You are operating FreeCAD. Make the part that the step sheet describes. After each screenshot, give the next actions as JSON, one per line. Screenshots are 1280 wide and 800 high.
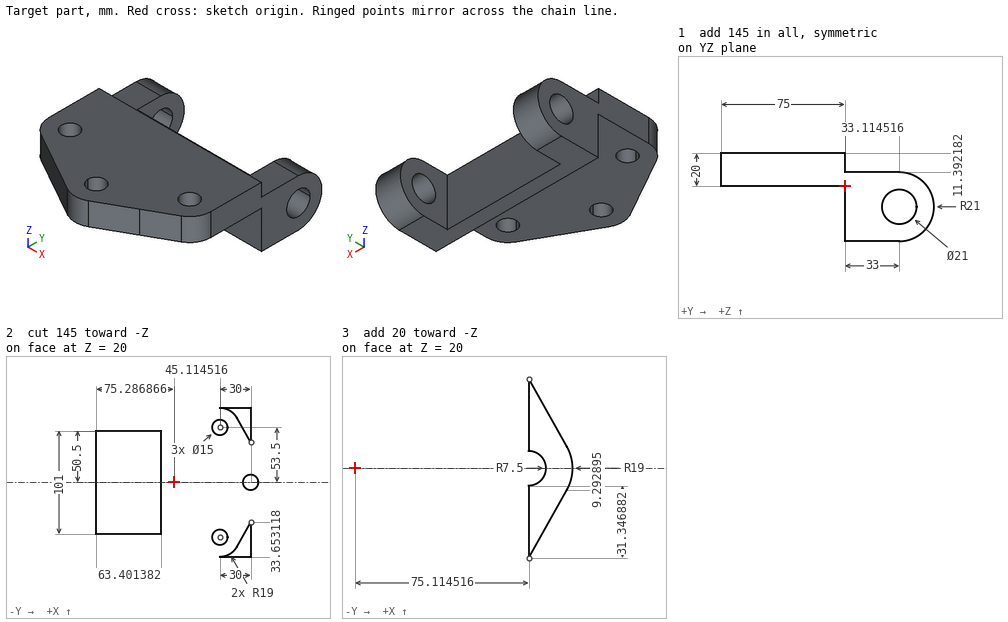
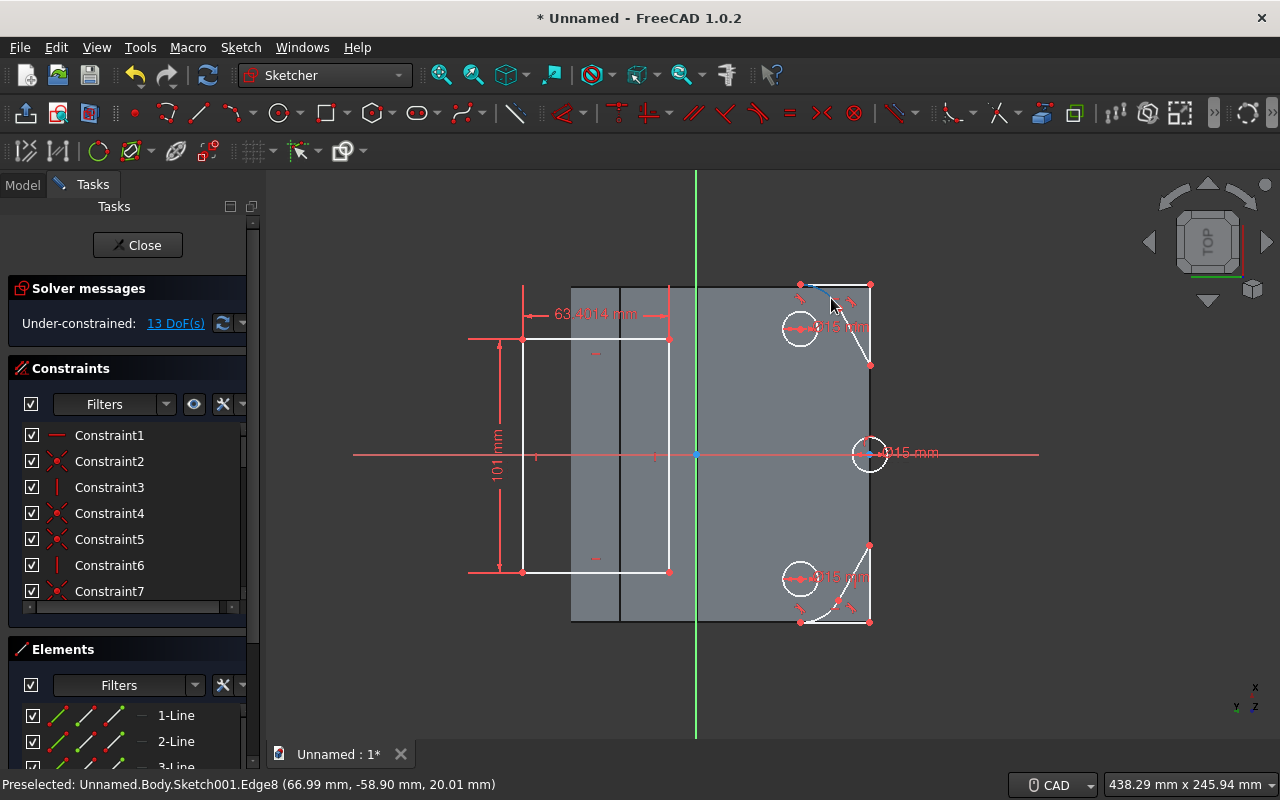
{"action": "scroll", "coordinate": [830, 611], "scroll_direction": "up", "scroll_amount": 4}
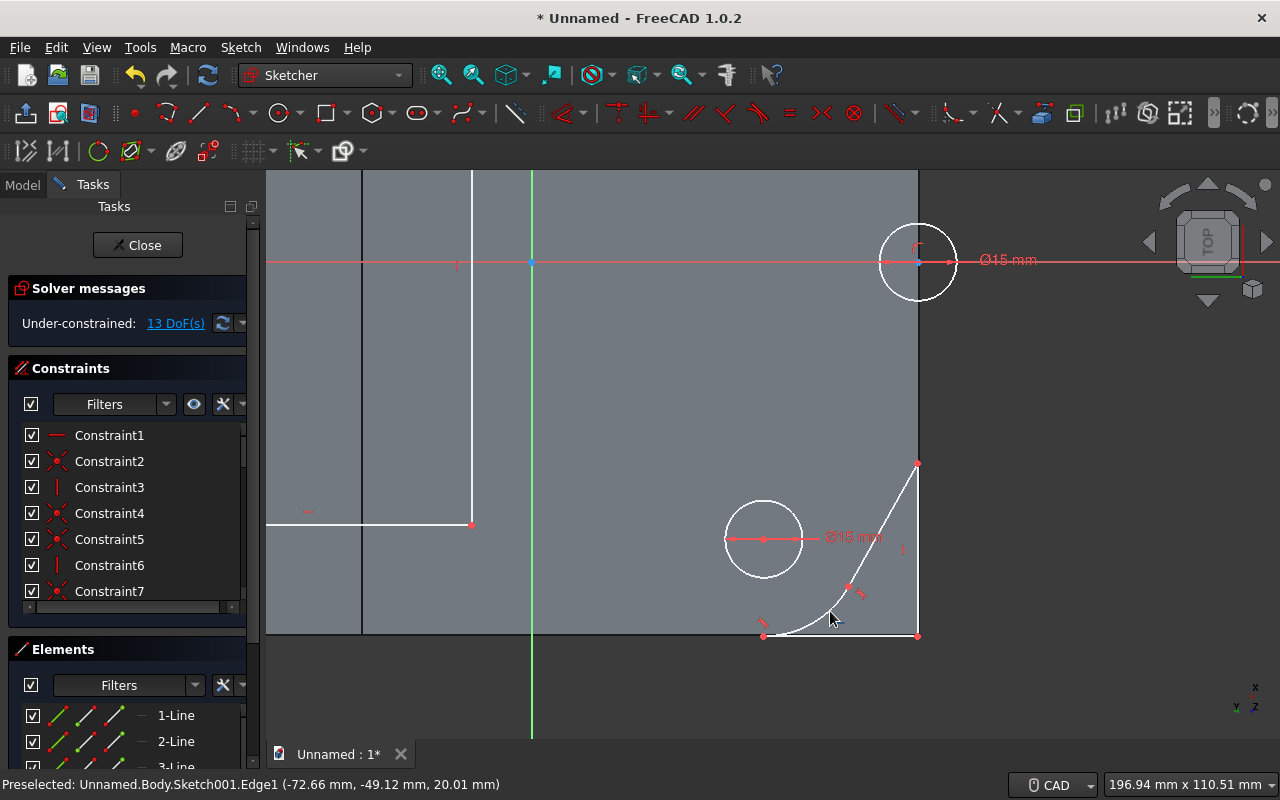
{"action": "left_click", "coordinate": [830, 611]}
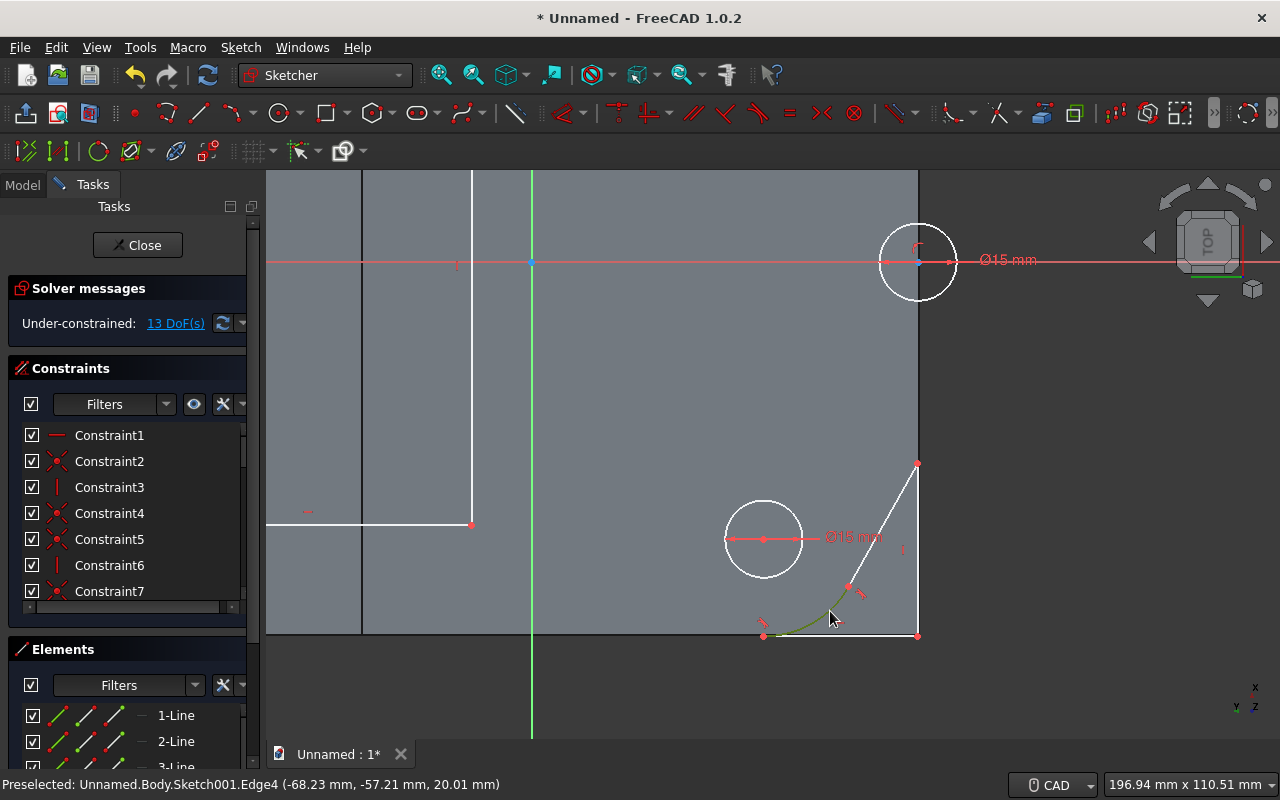
{"action": "scroll", "coordinate": [830, 611], "scroll_direction": "down", "scroll_amount": 4}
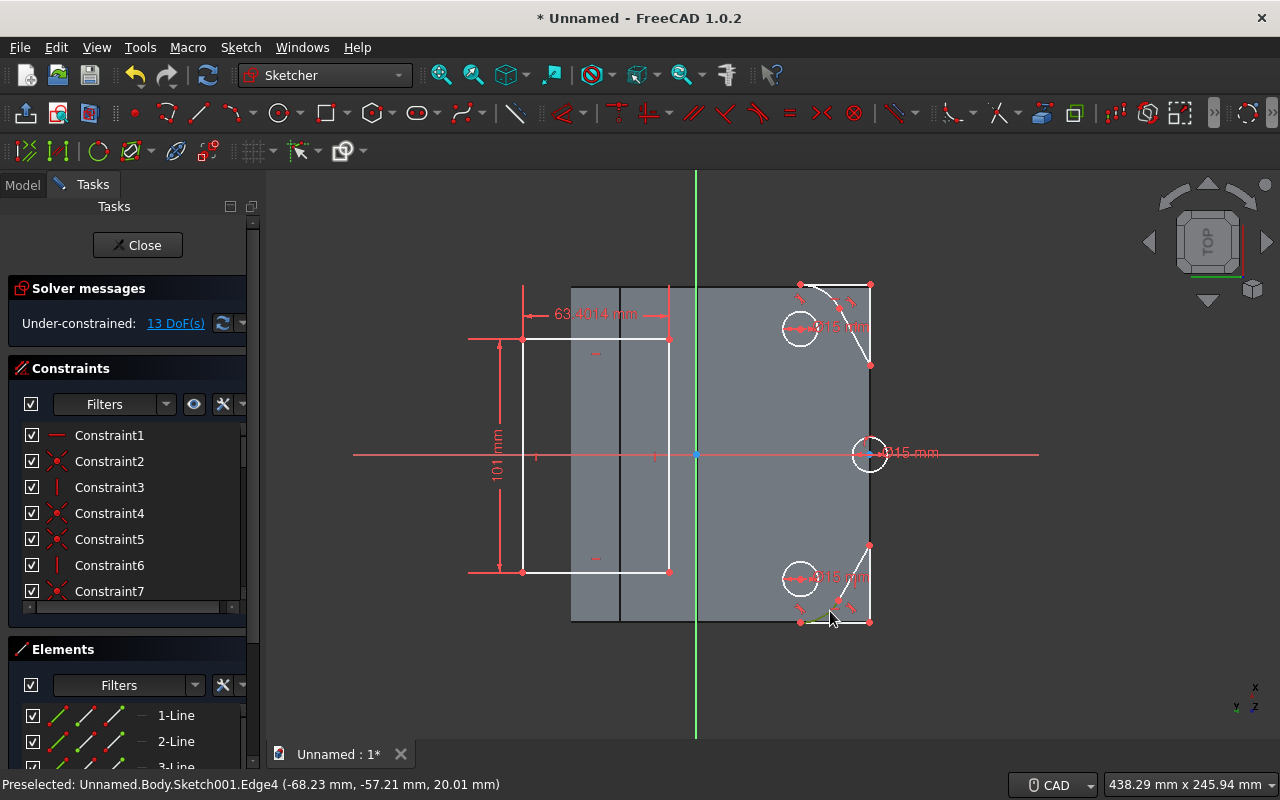
{"action": "left_click", "coordinate": [823, 291]}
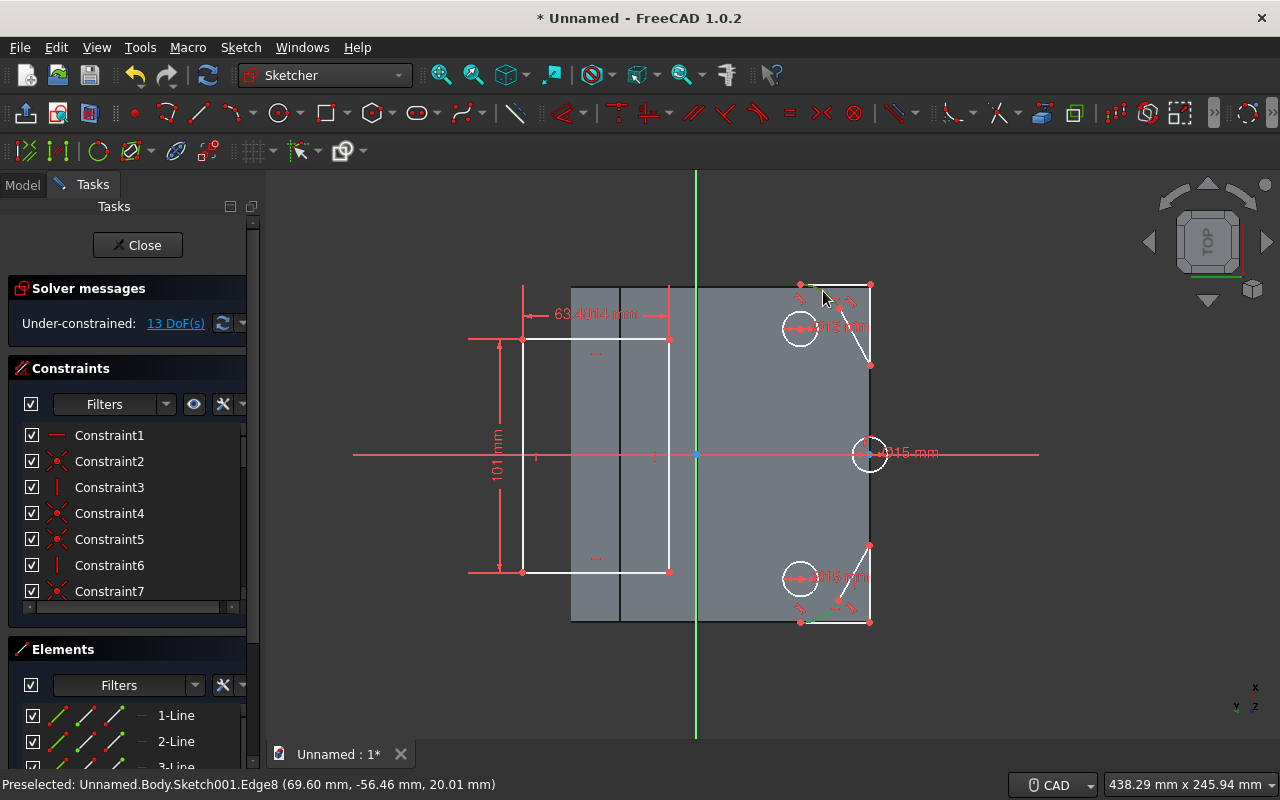
{"action": "left_click", "coordinate": [790, 114]}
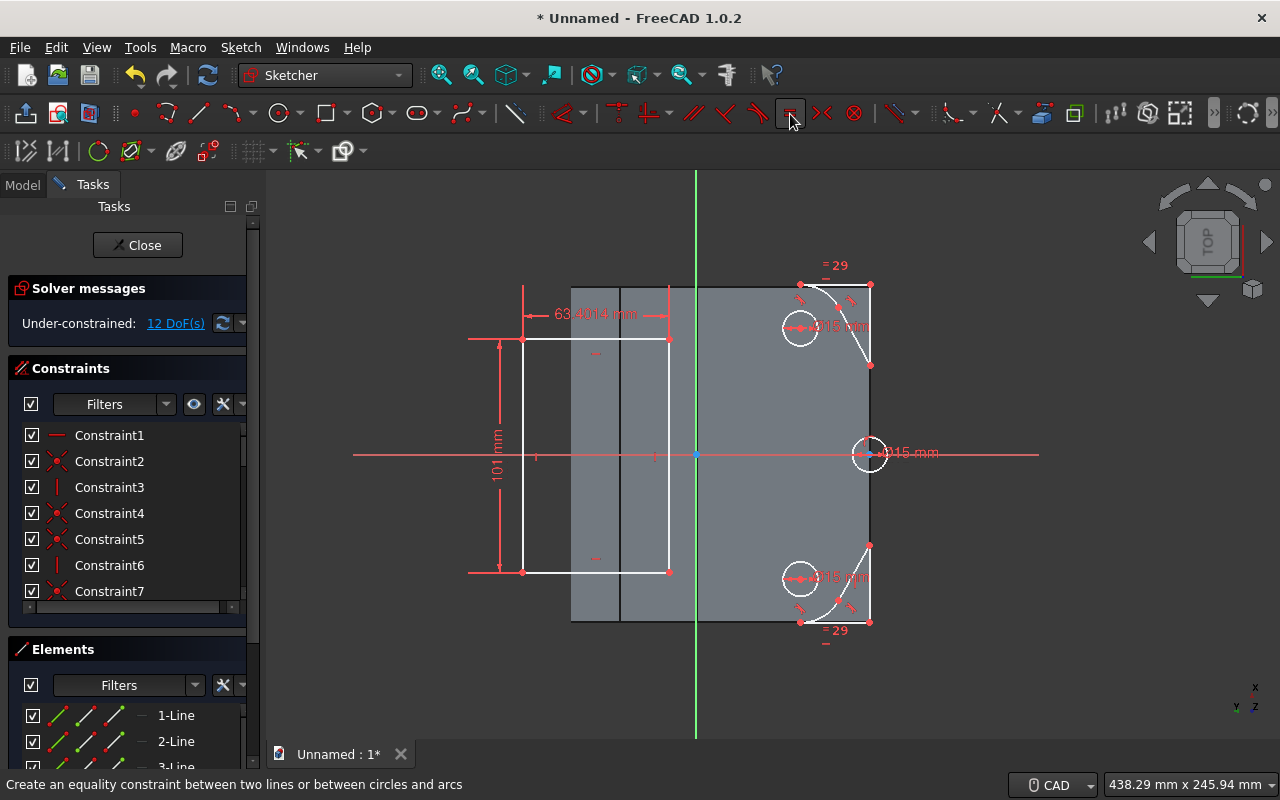
{"action": "left_click", "coordinate": [801, 579]}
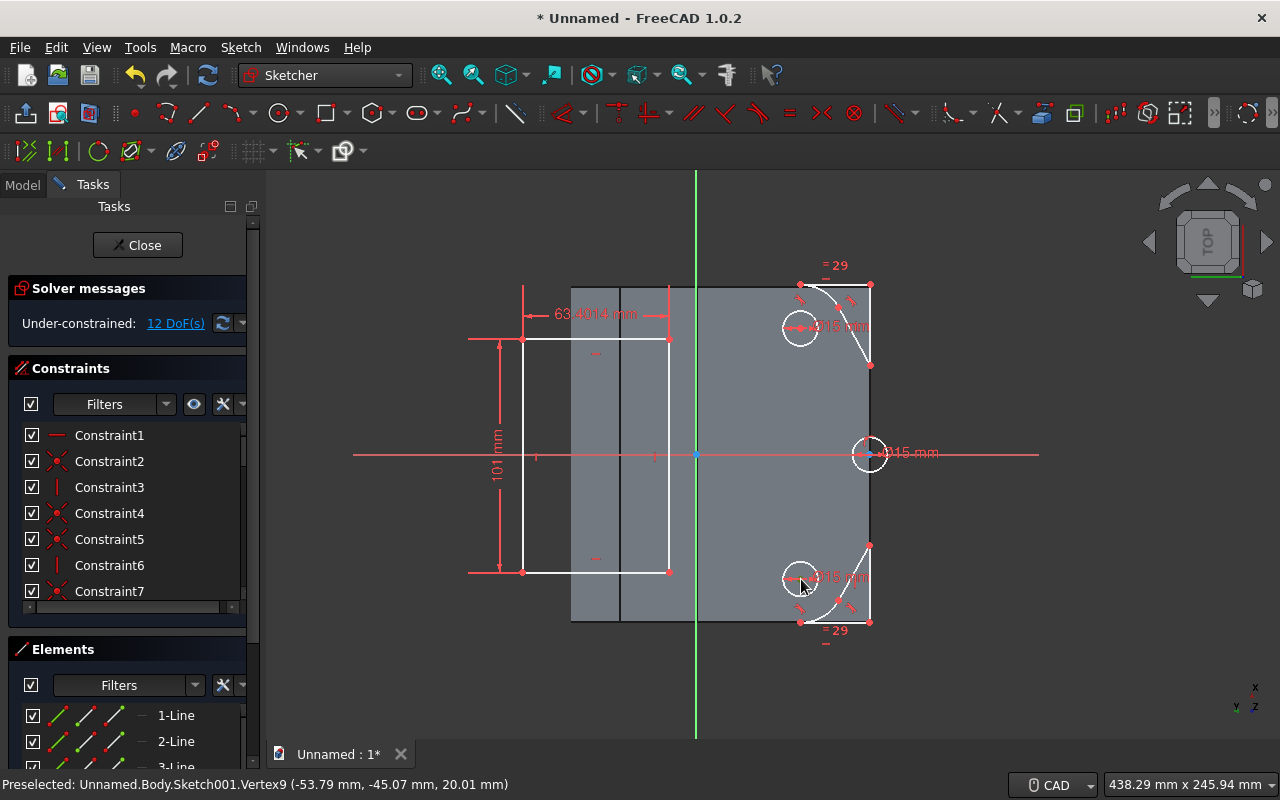
{"action": "left_click", "coordinate": [800, 328]}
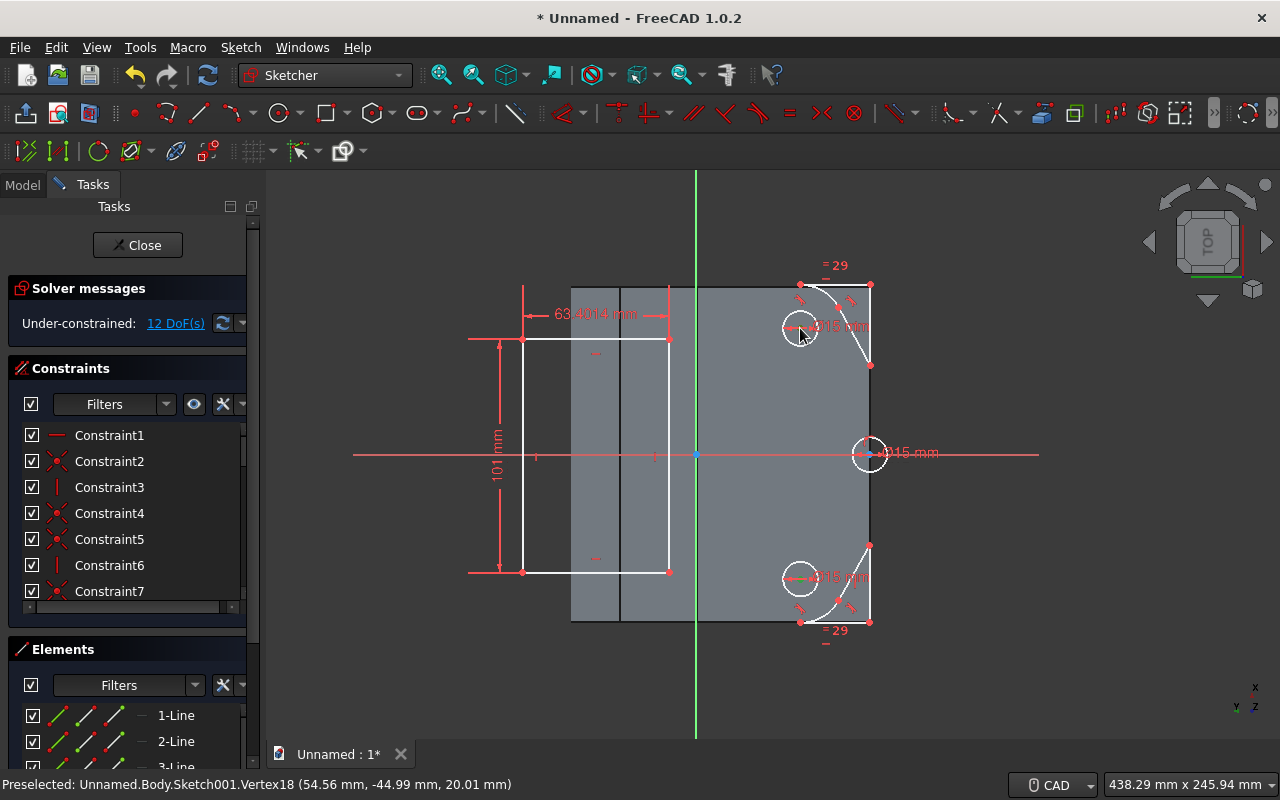
{"action": "left_click", "coordinate": [353, 455]}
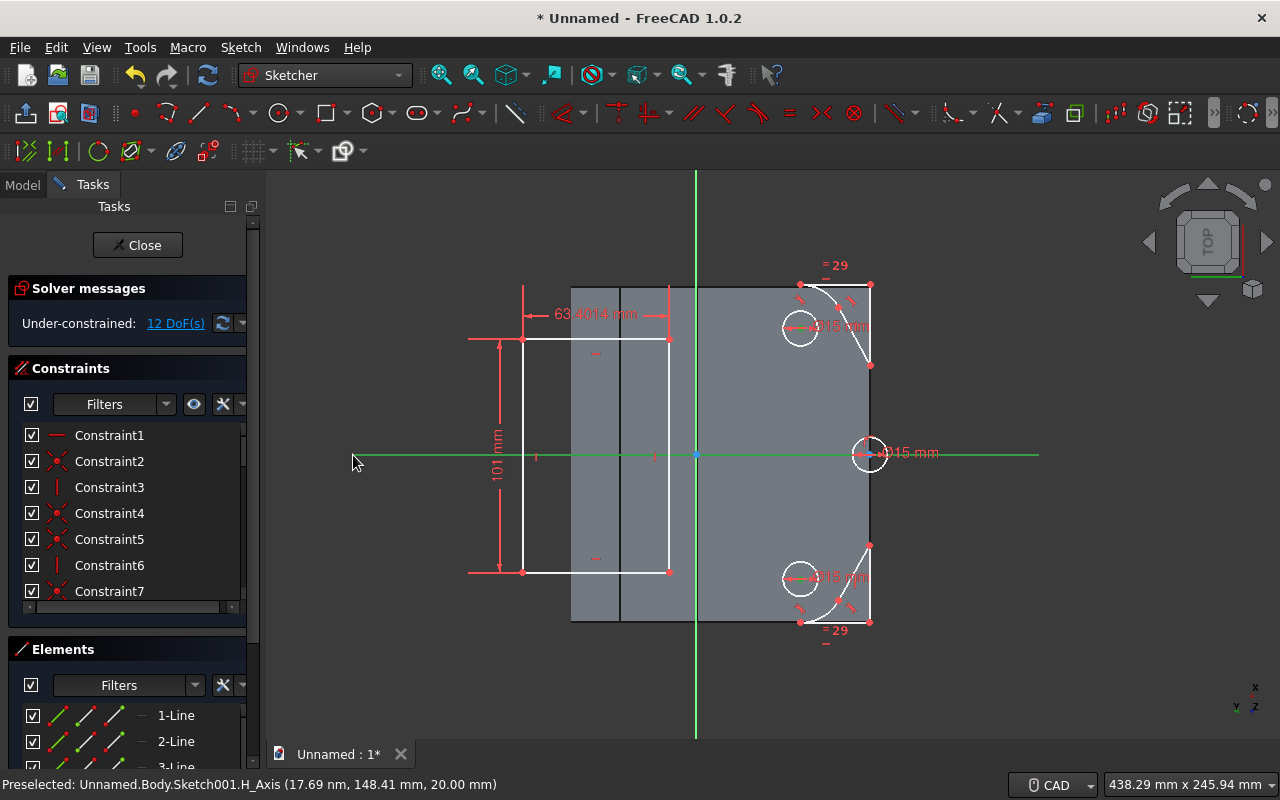
{"action": "left_click", "coordinate": [822, 114]}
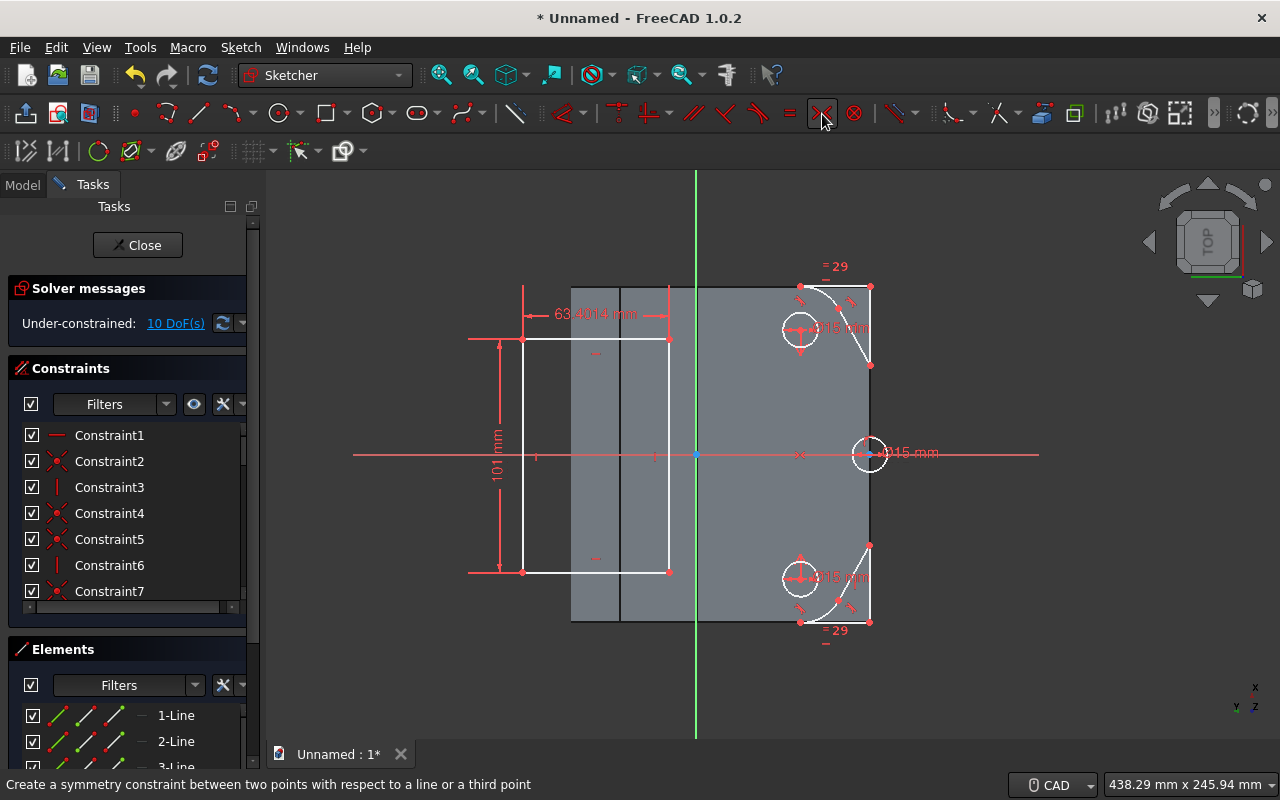
{"action": "left_click", "coordinate": [870, 545]}